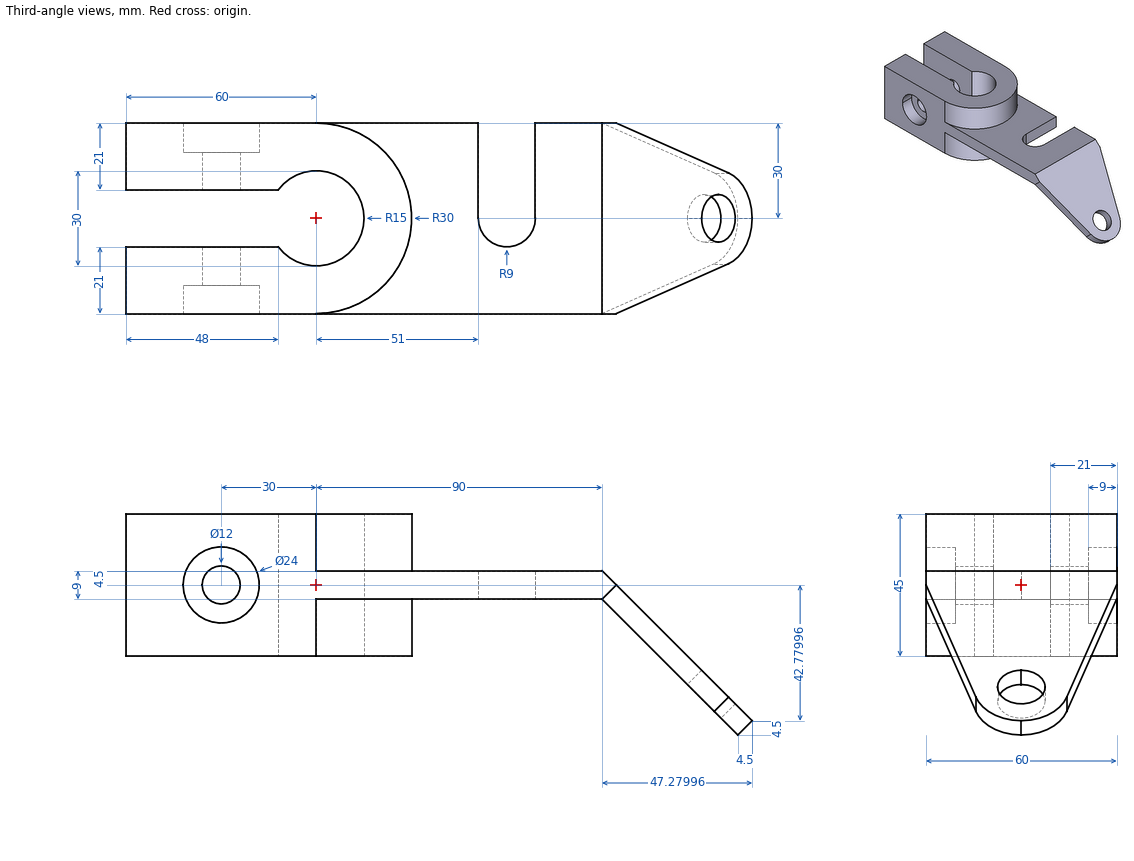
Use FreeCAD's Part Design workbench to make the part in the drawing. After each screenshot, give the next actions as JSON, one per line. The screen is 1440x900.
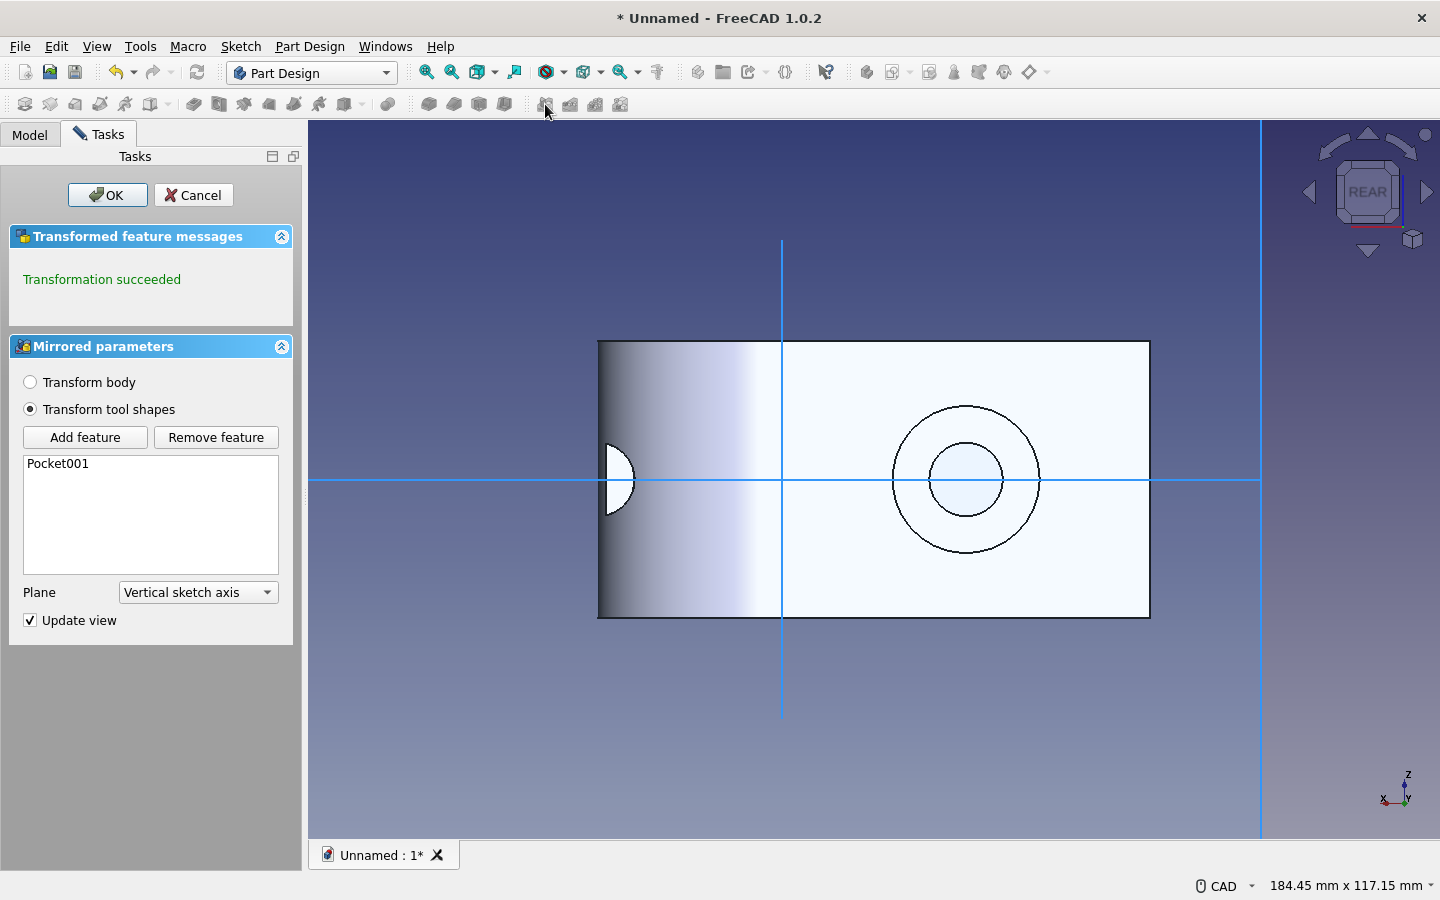
{"action": "left_click", "coordinate": [199, 592]}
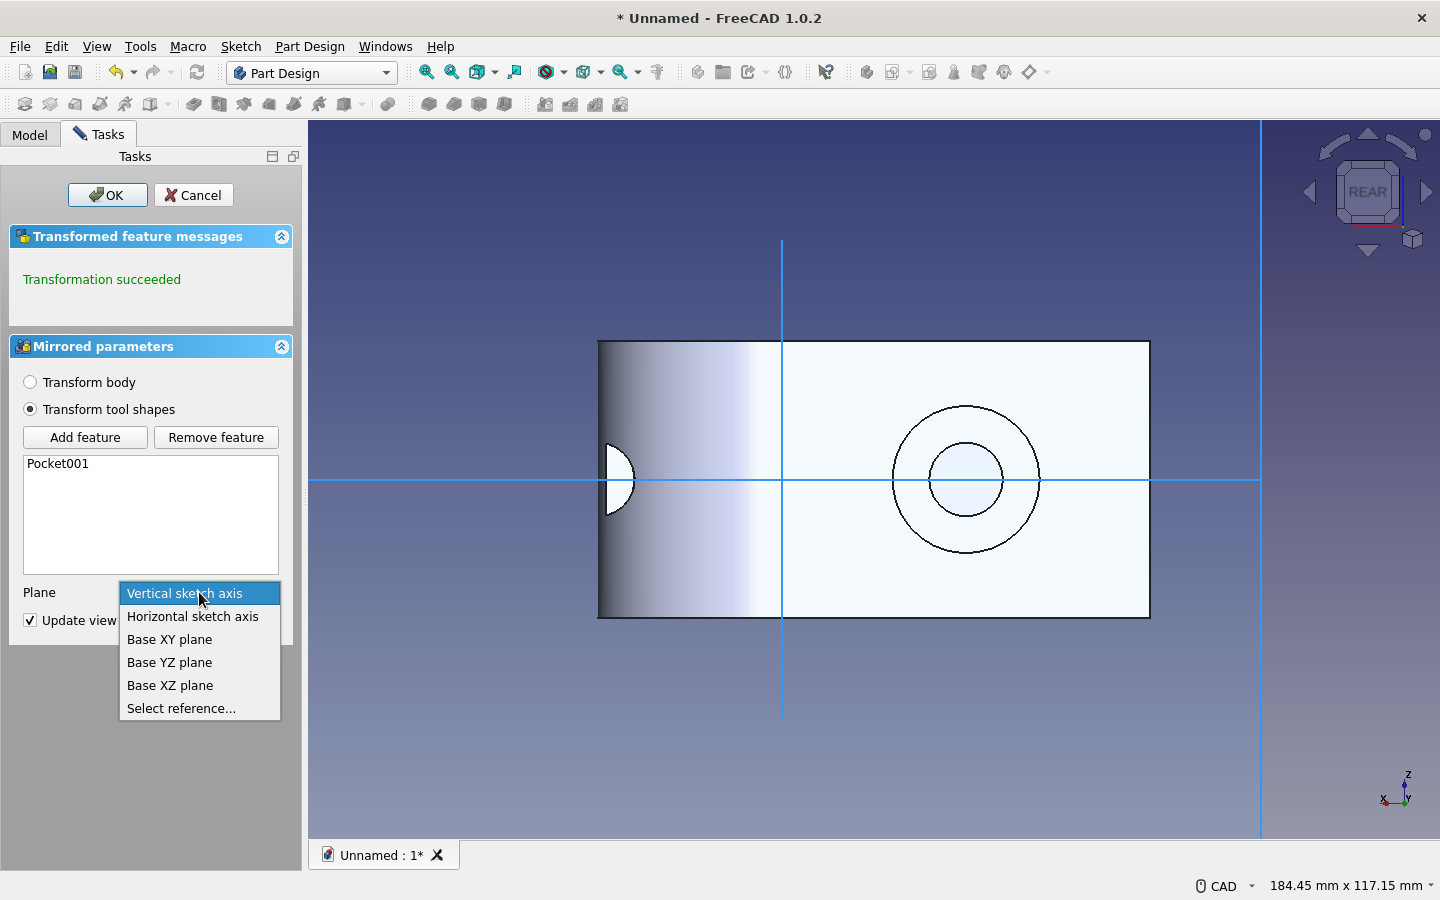
{"action": "left_click", "coordinate": [198, 686]}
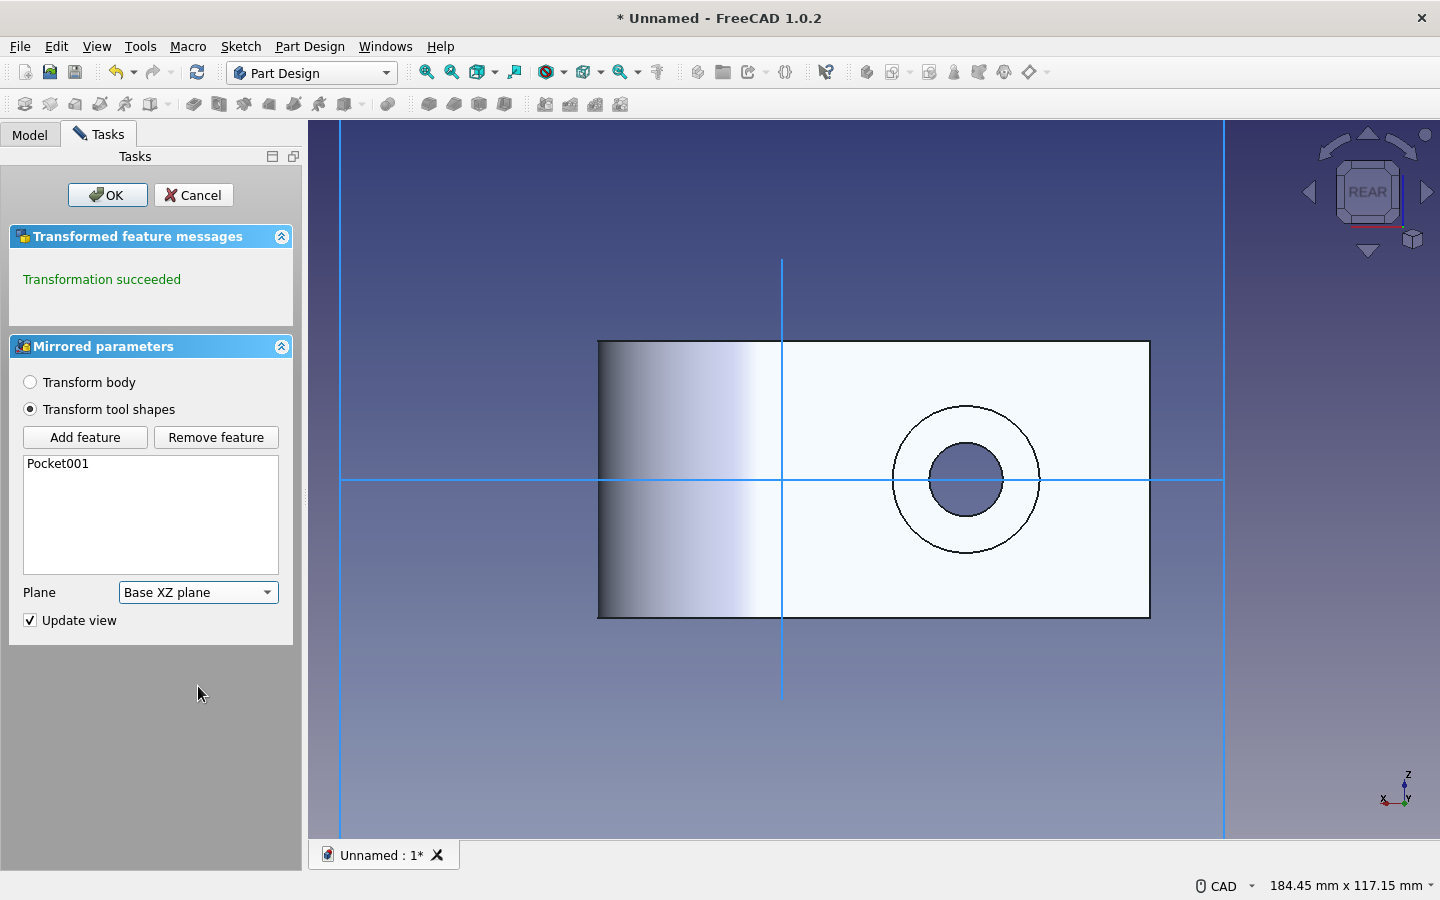
{"action": "left_click", "coordinate": [108, 195]}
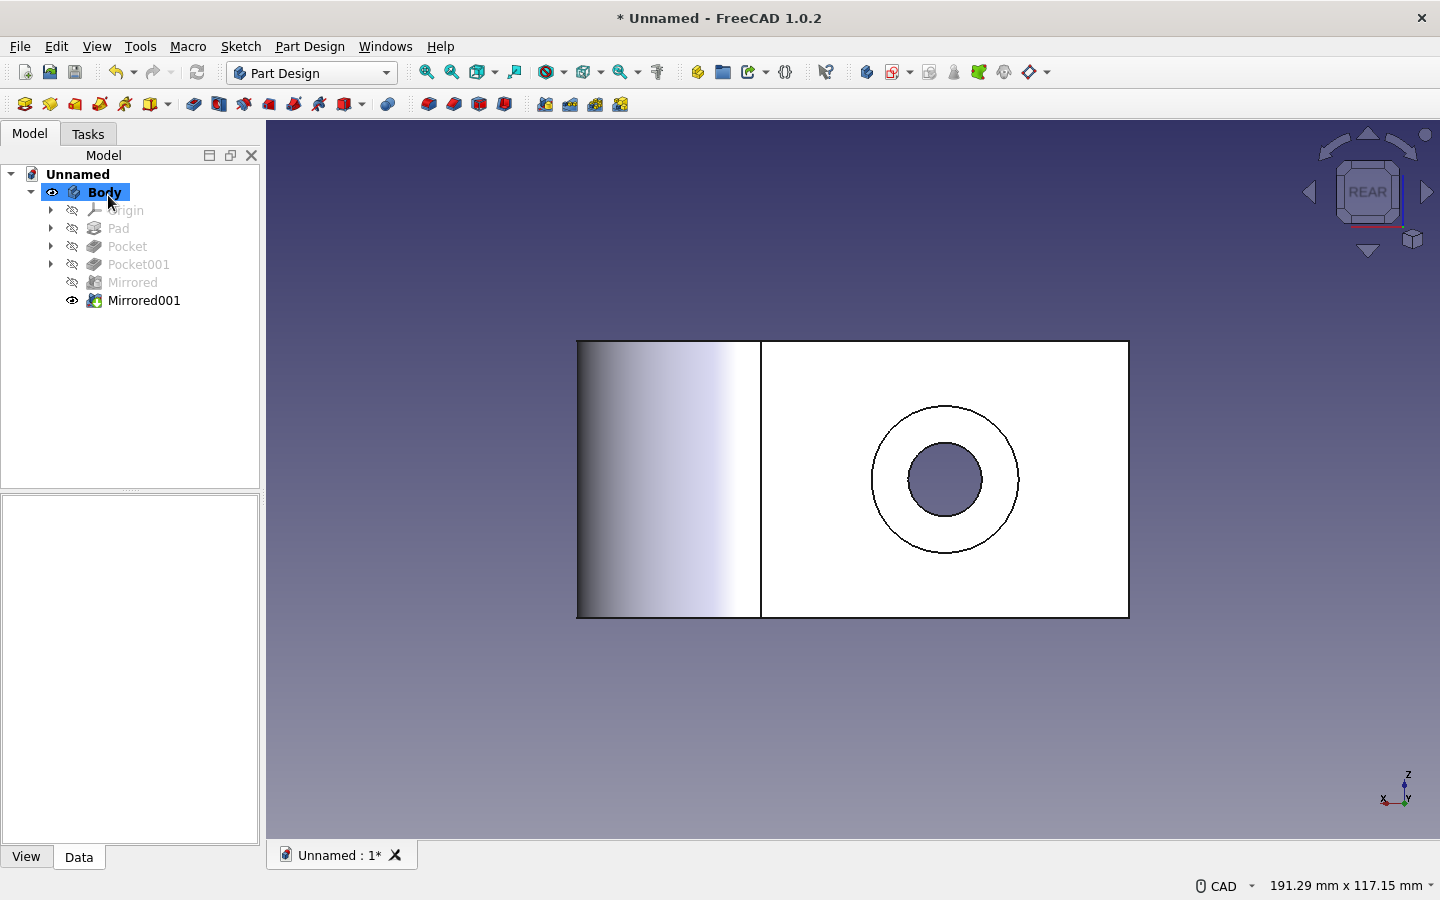
{"action": "left_click", "coordinate": [892, 72]}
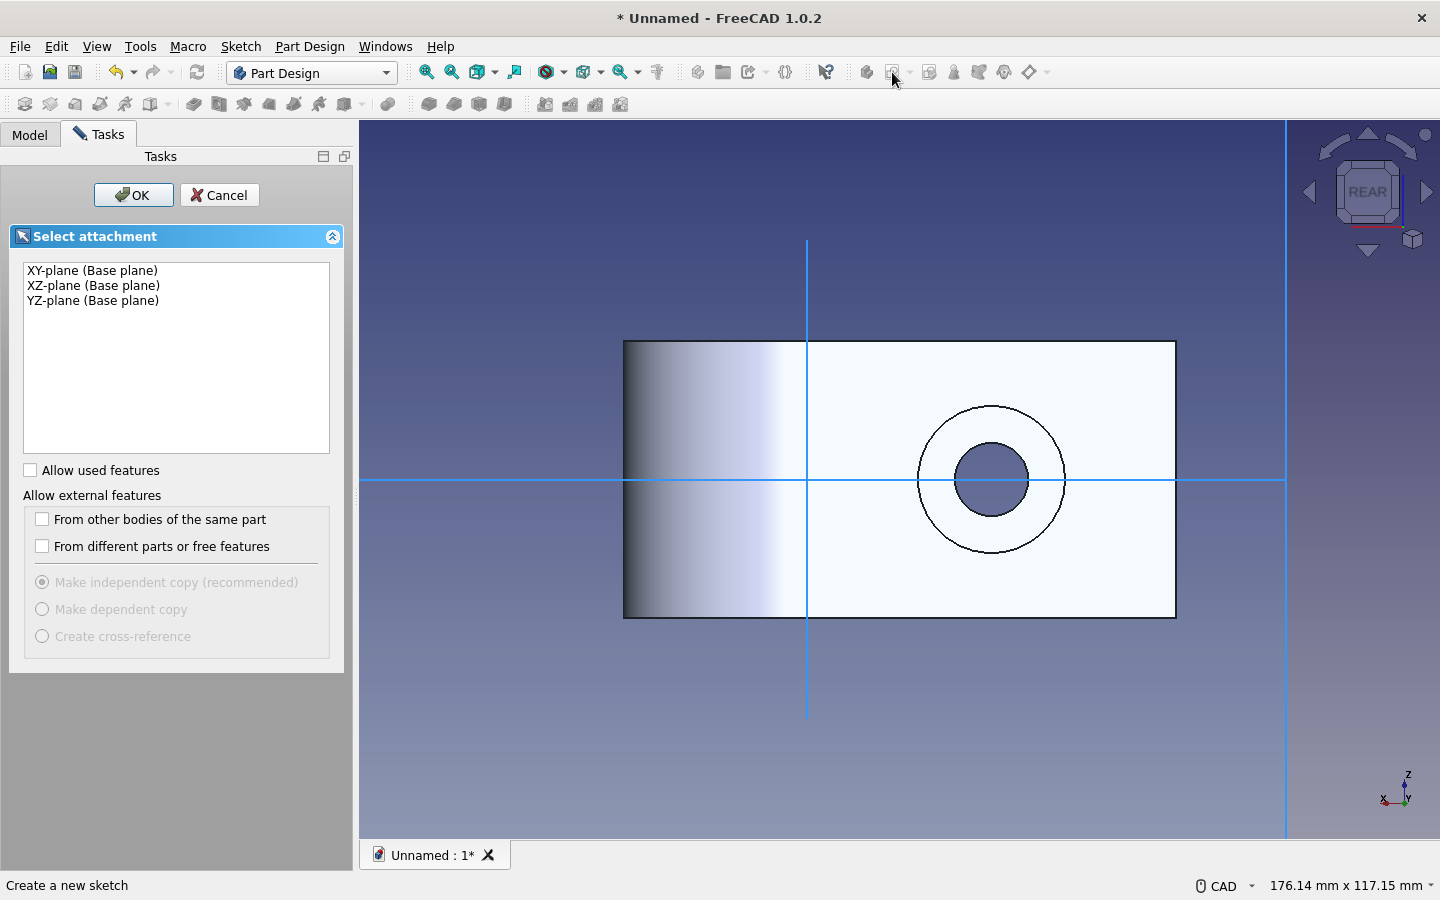
{"action": "left_click", "coordinate": [84, 286]}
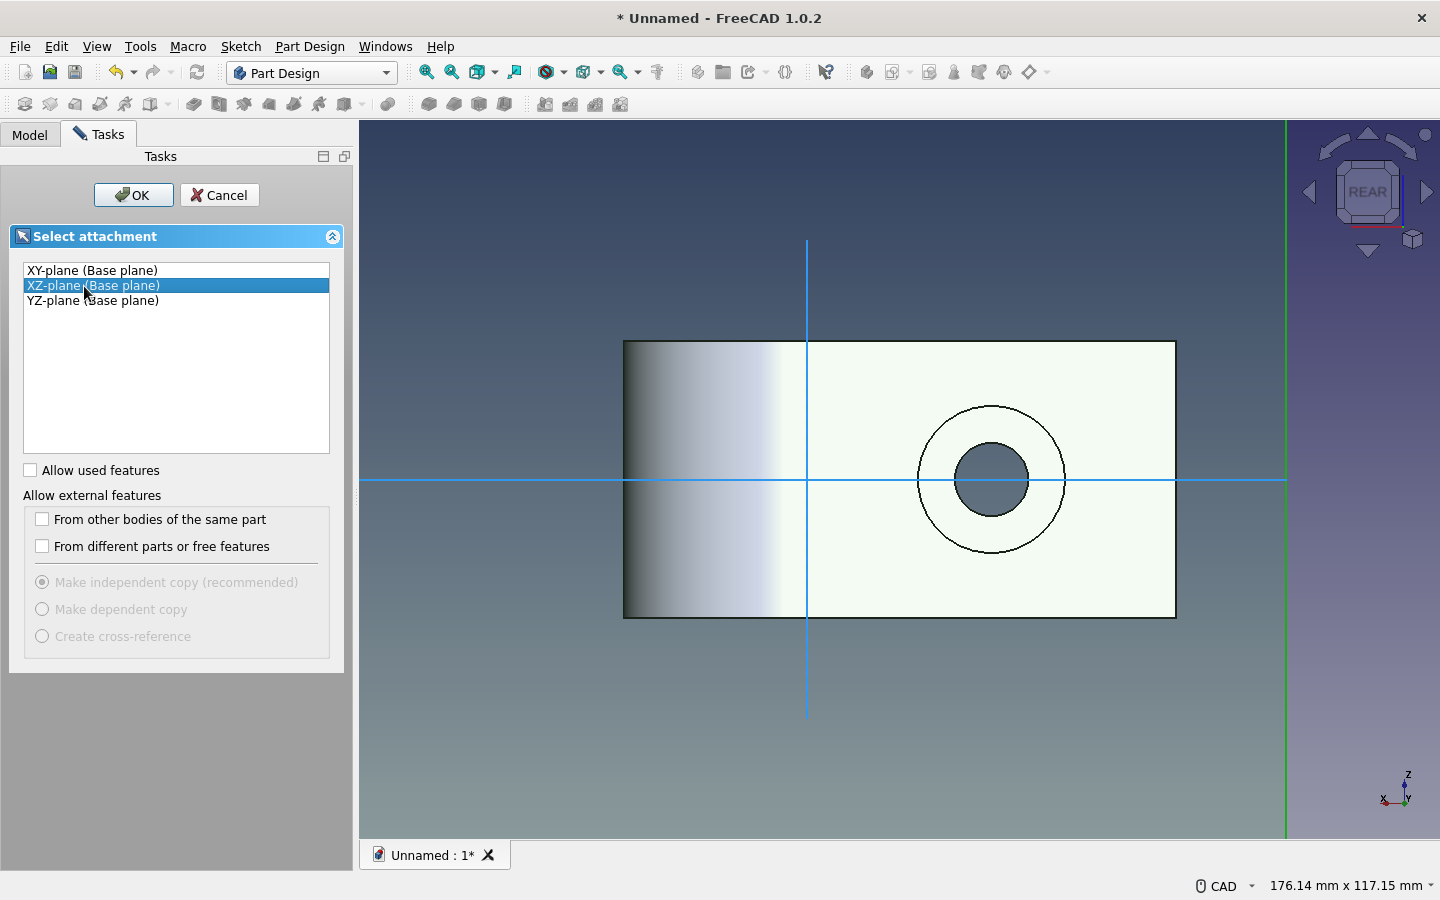
{"action": "left_click", "coordinate": [134, 195]}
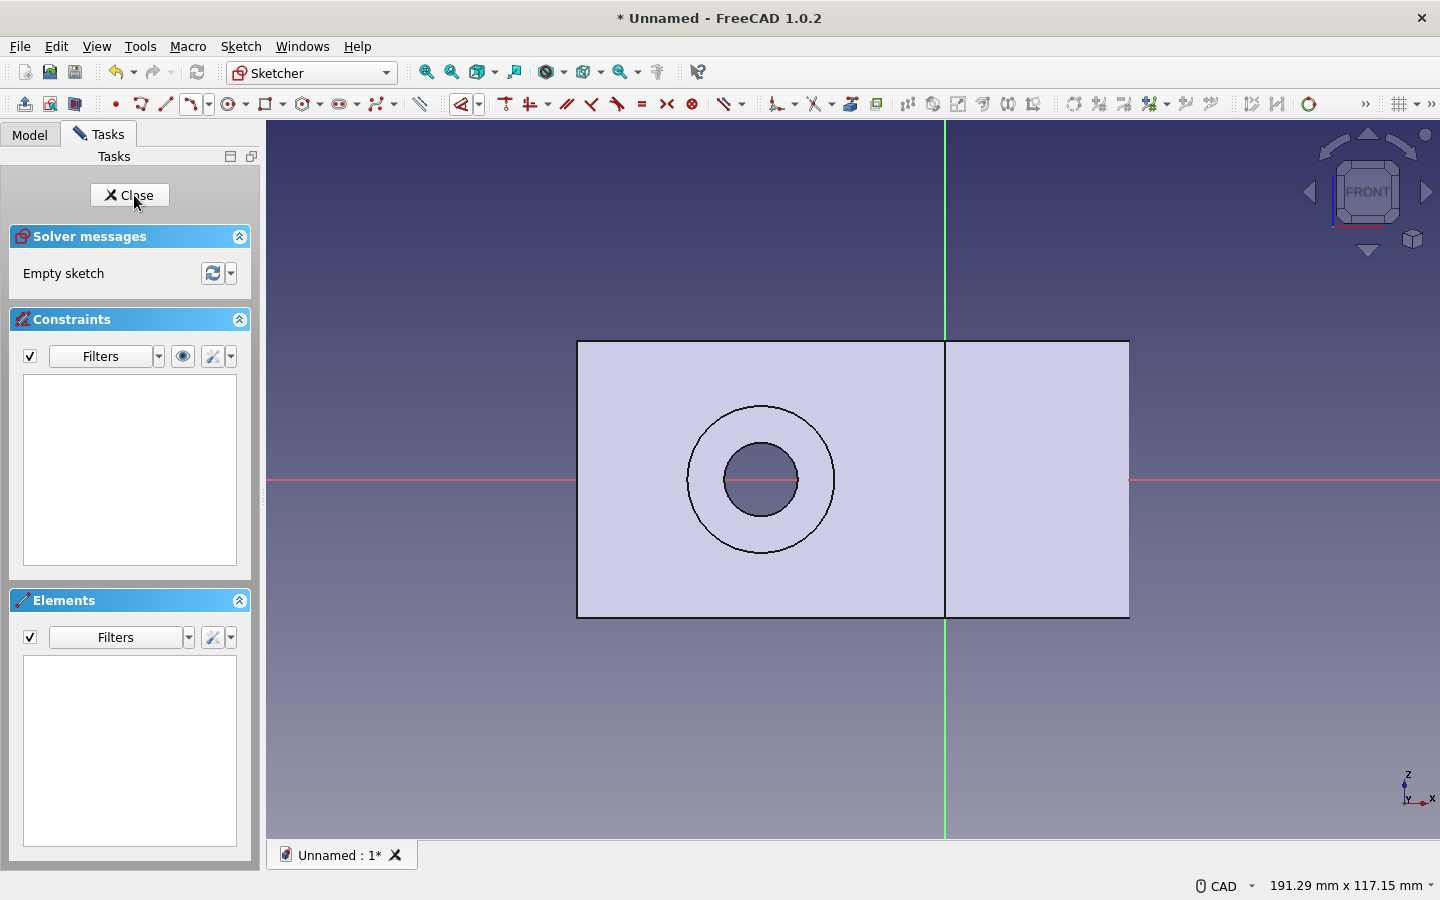
{"action": "key", "text": "q s"}